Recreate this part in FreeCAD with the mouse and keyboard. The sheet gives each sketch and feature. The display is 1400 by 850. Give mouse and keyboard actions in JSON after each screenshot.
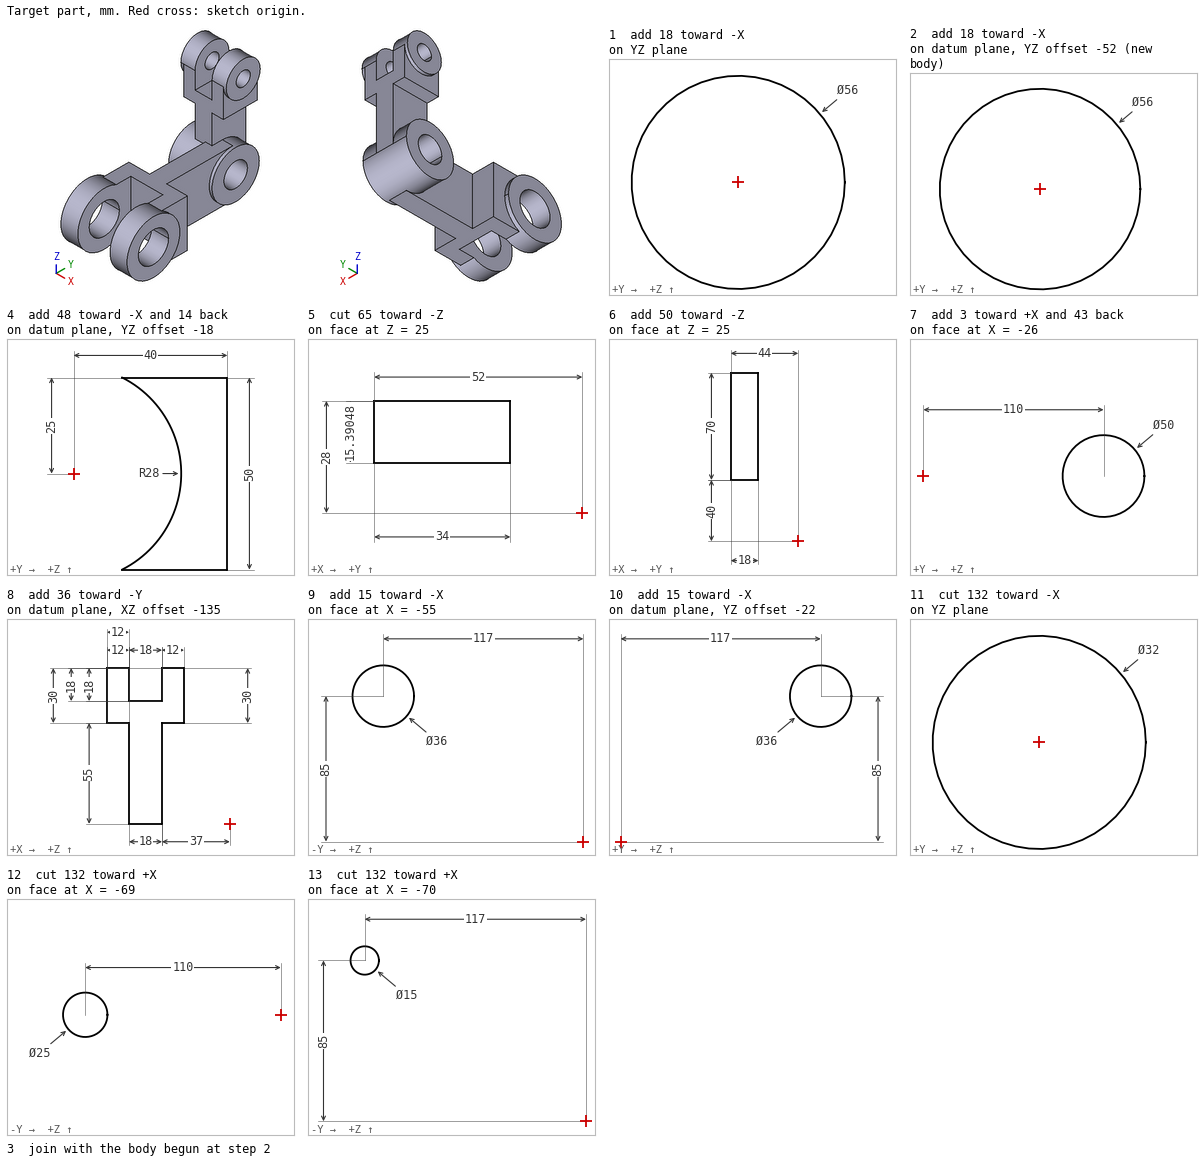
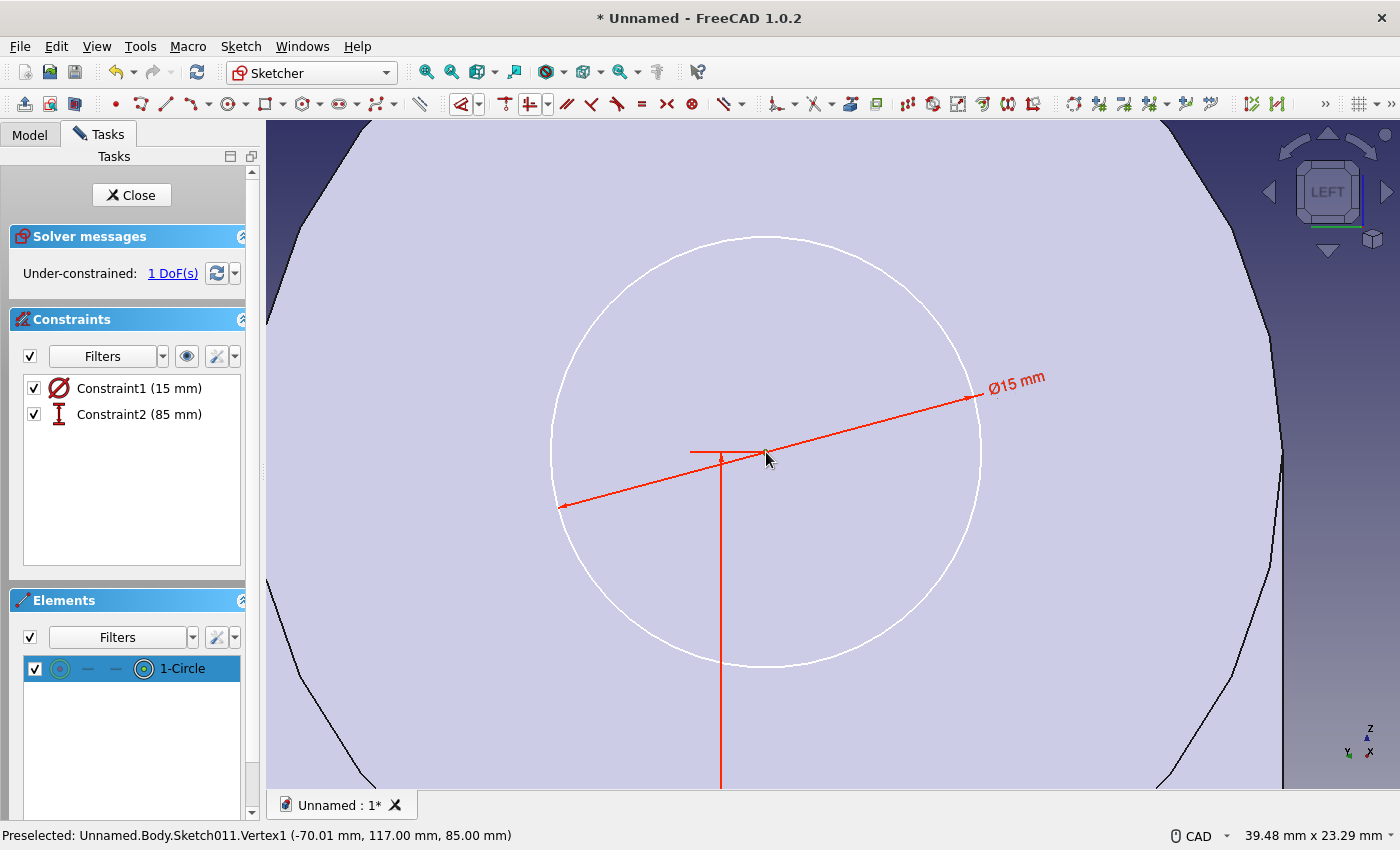
{"action": "key", "text": "l"}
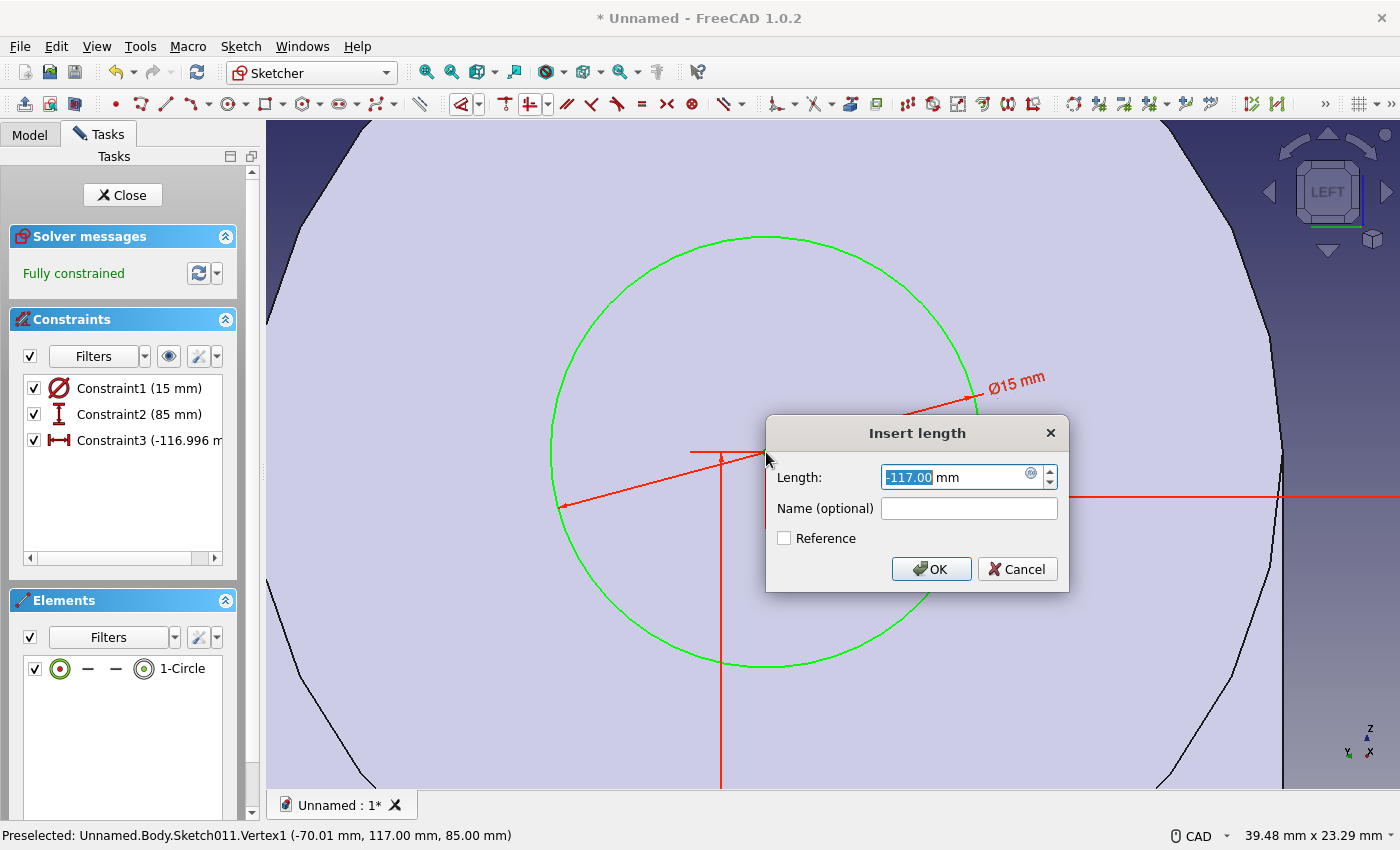
{"action": "type", "text": "-117"}
{"action": "key", "text": "Return"}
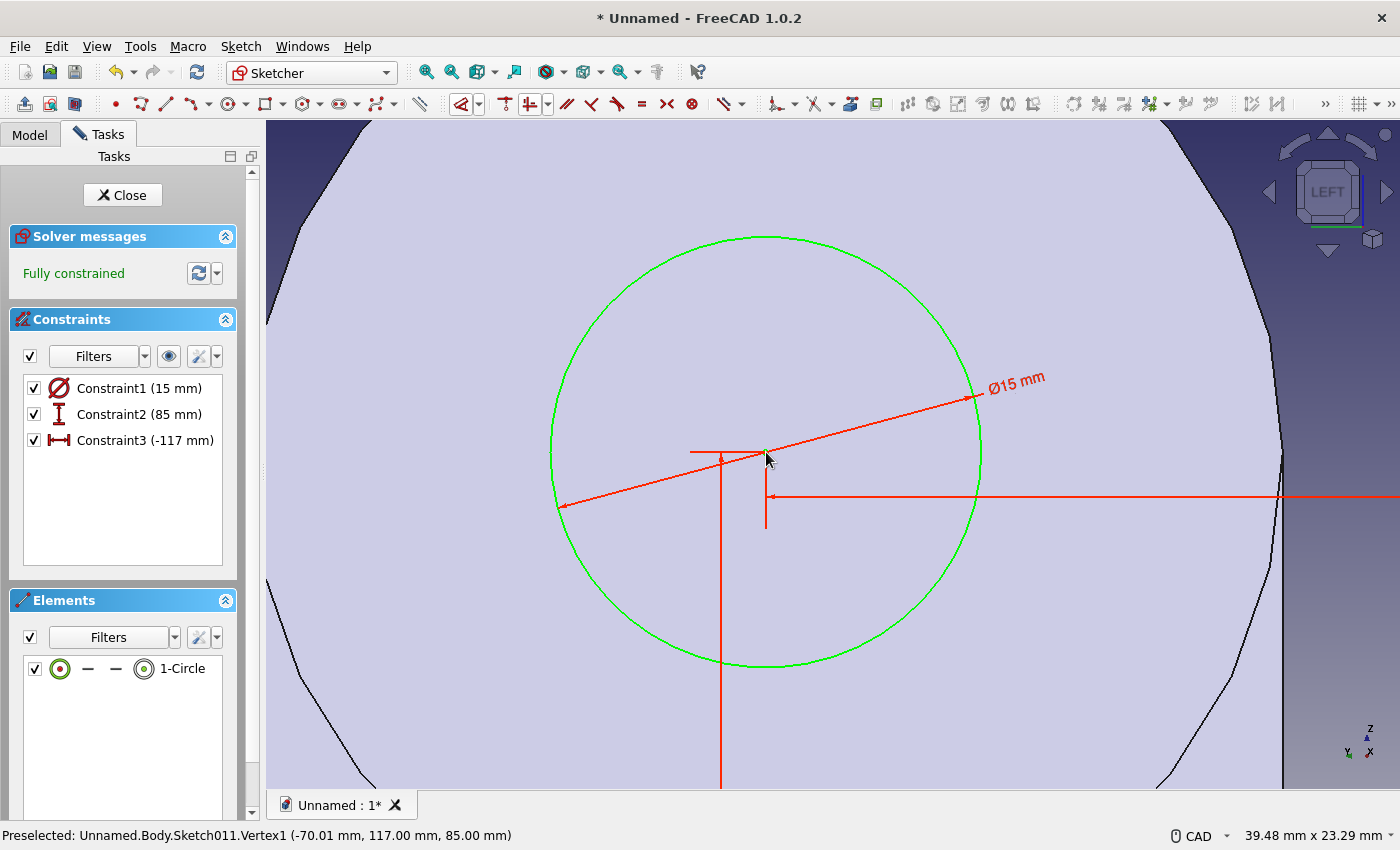
{"action": "left_click", "coordinate": [123, 195]}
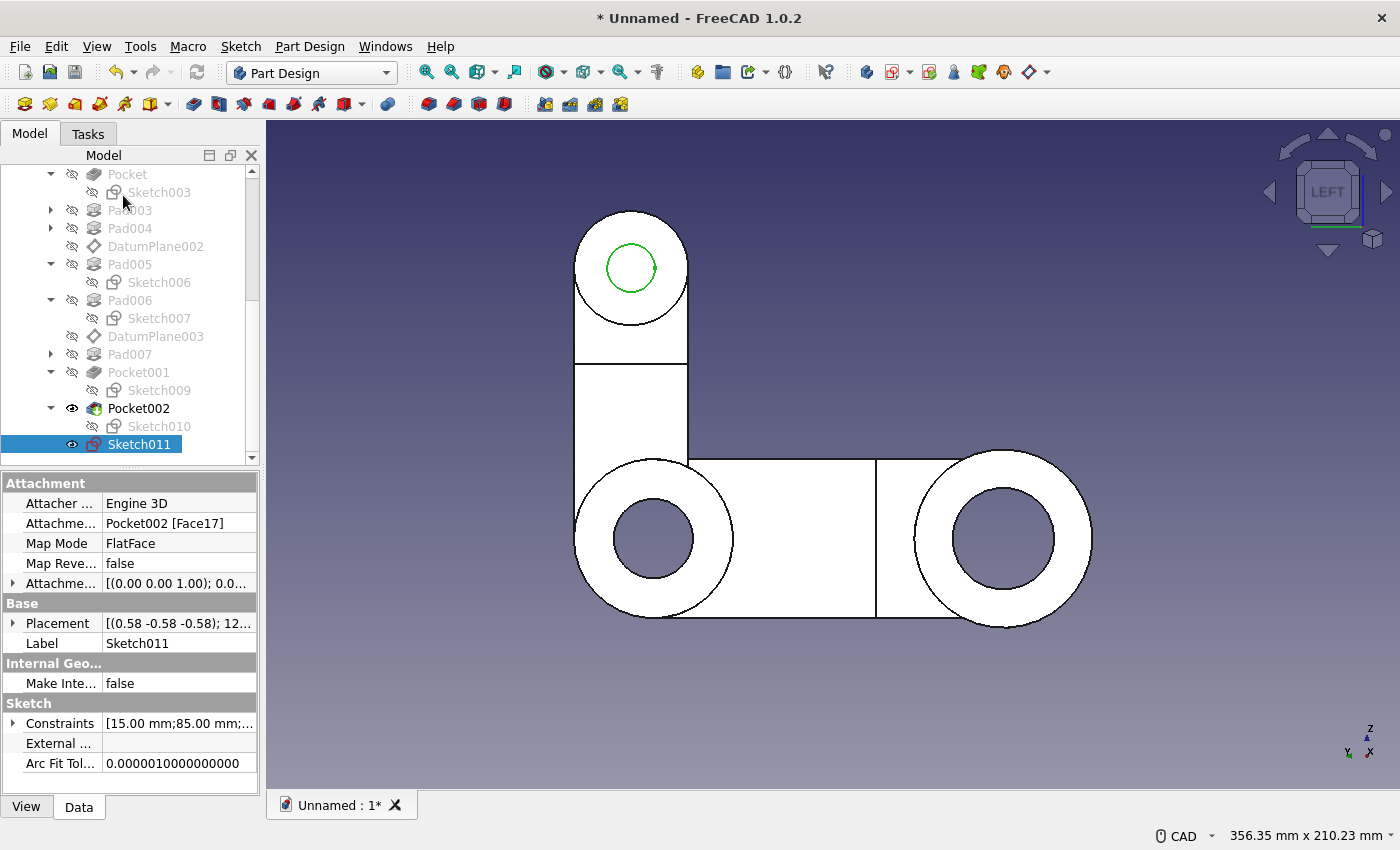
{"action": "left_click", "coordinate": [194, 104]}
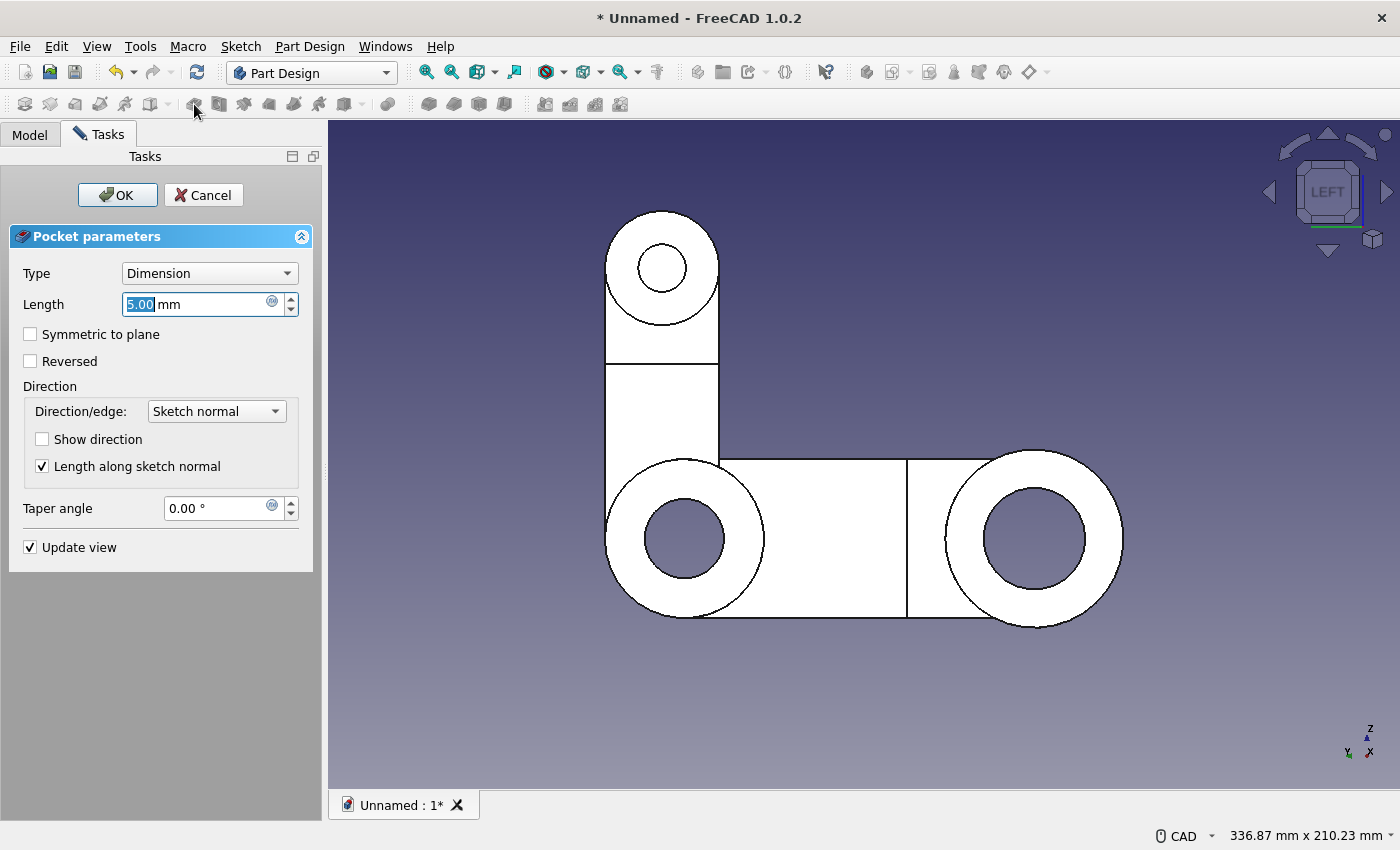
{"action": "type", "text": "132"}
{"action": "key", "text": "Tab"}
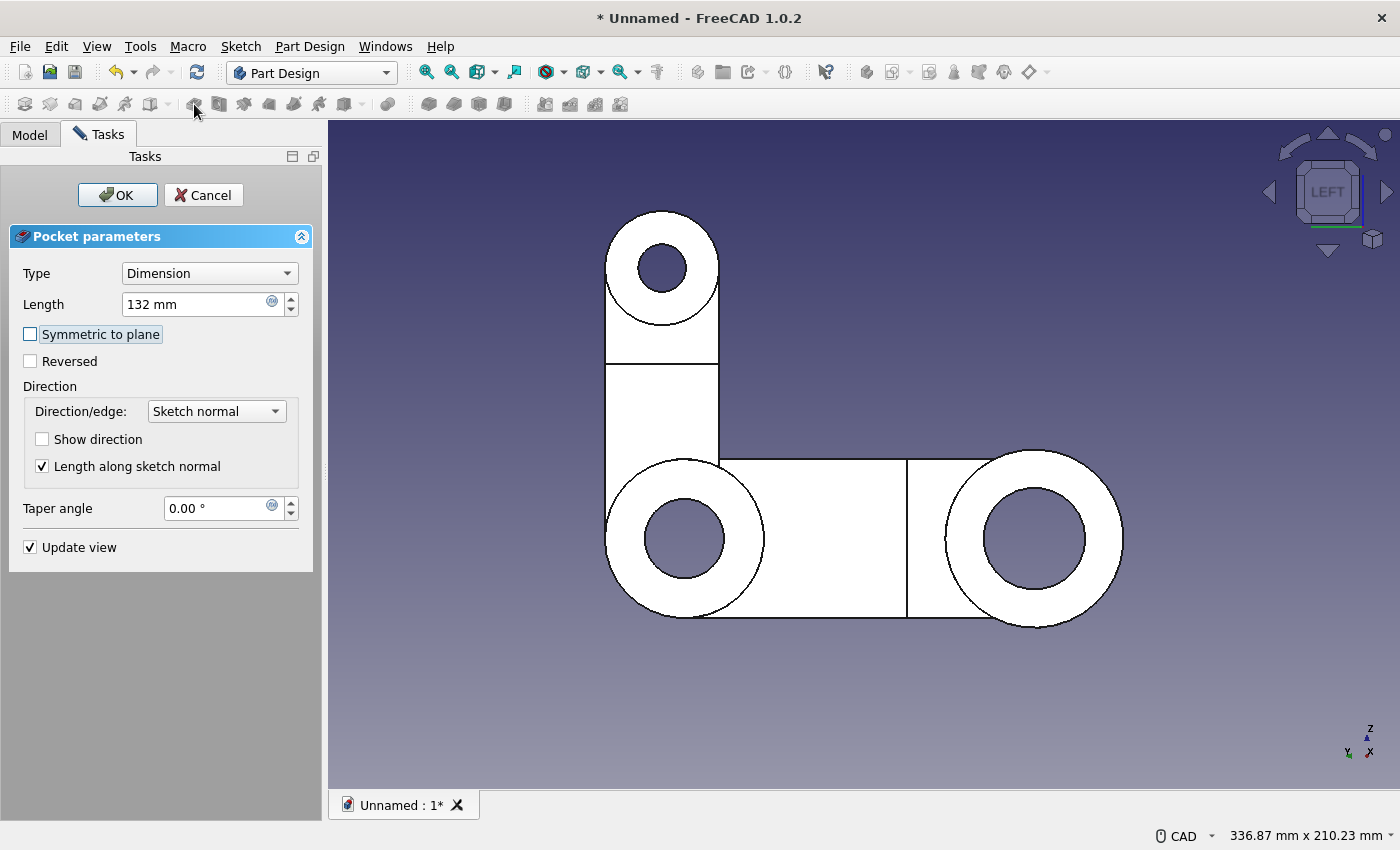
{"action": "left_click", "coordinate": [118, 195]}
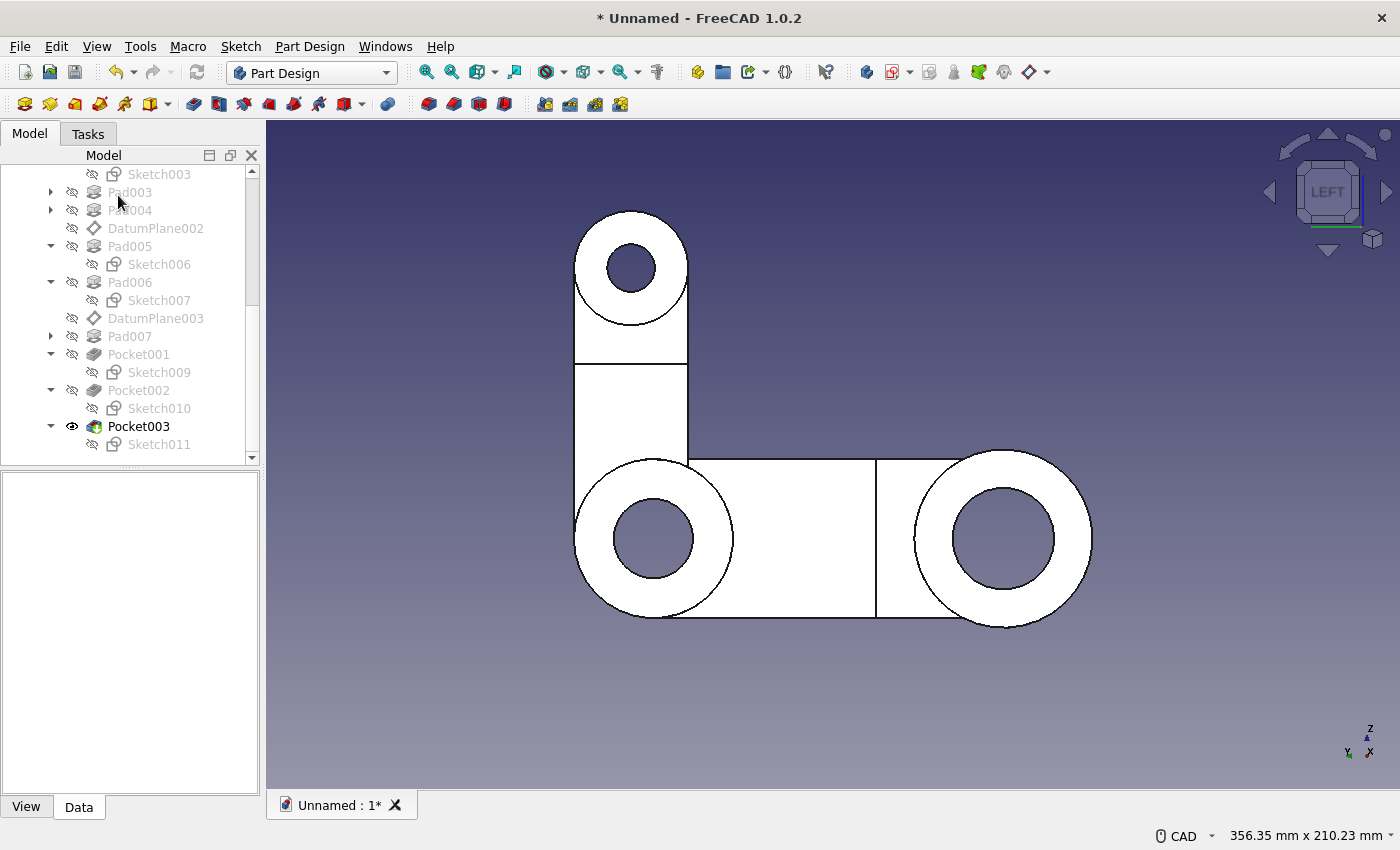
{"action": "key", "text": "0"}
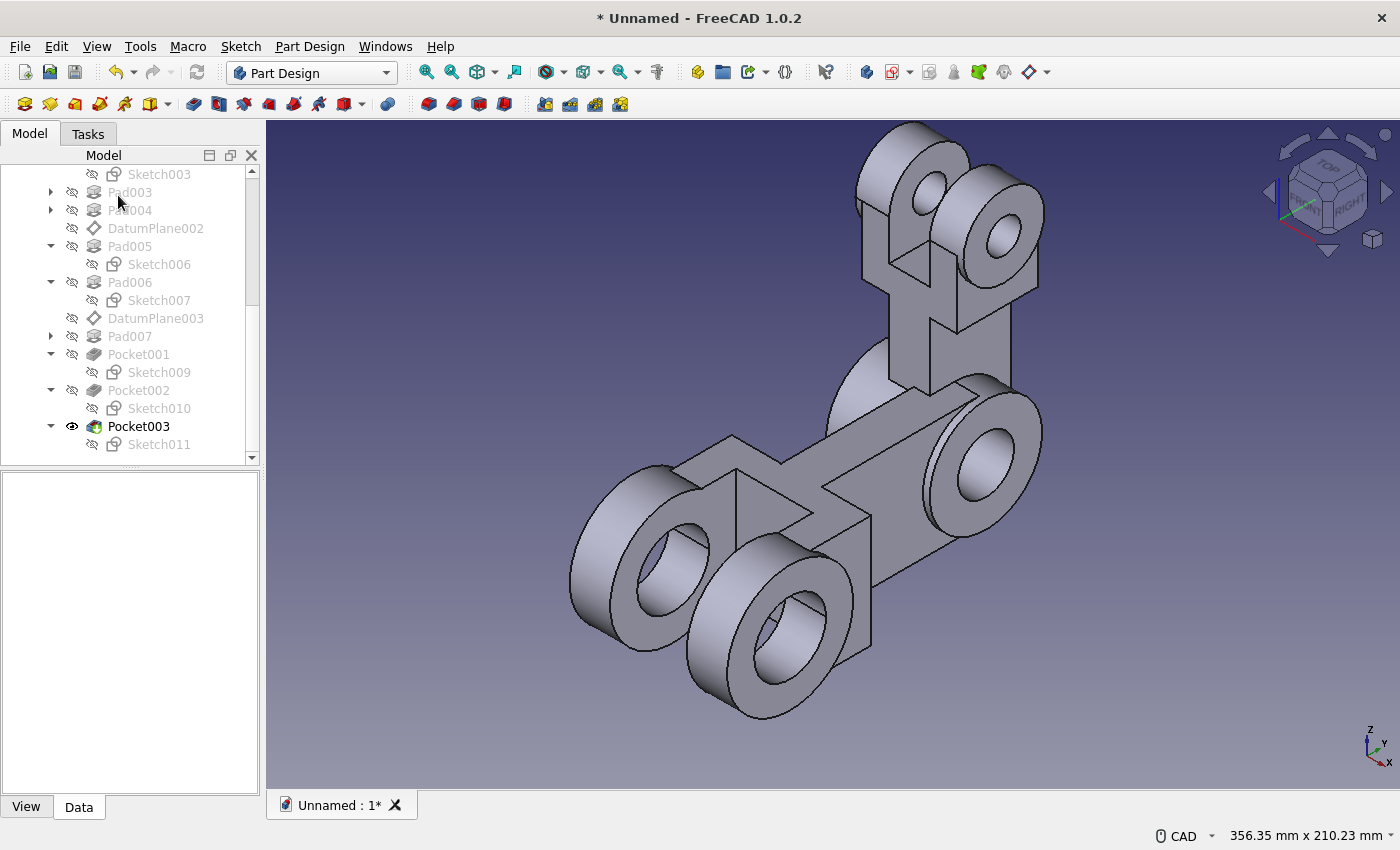
{"action": "left_click", "coordinate": [427, 72]}